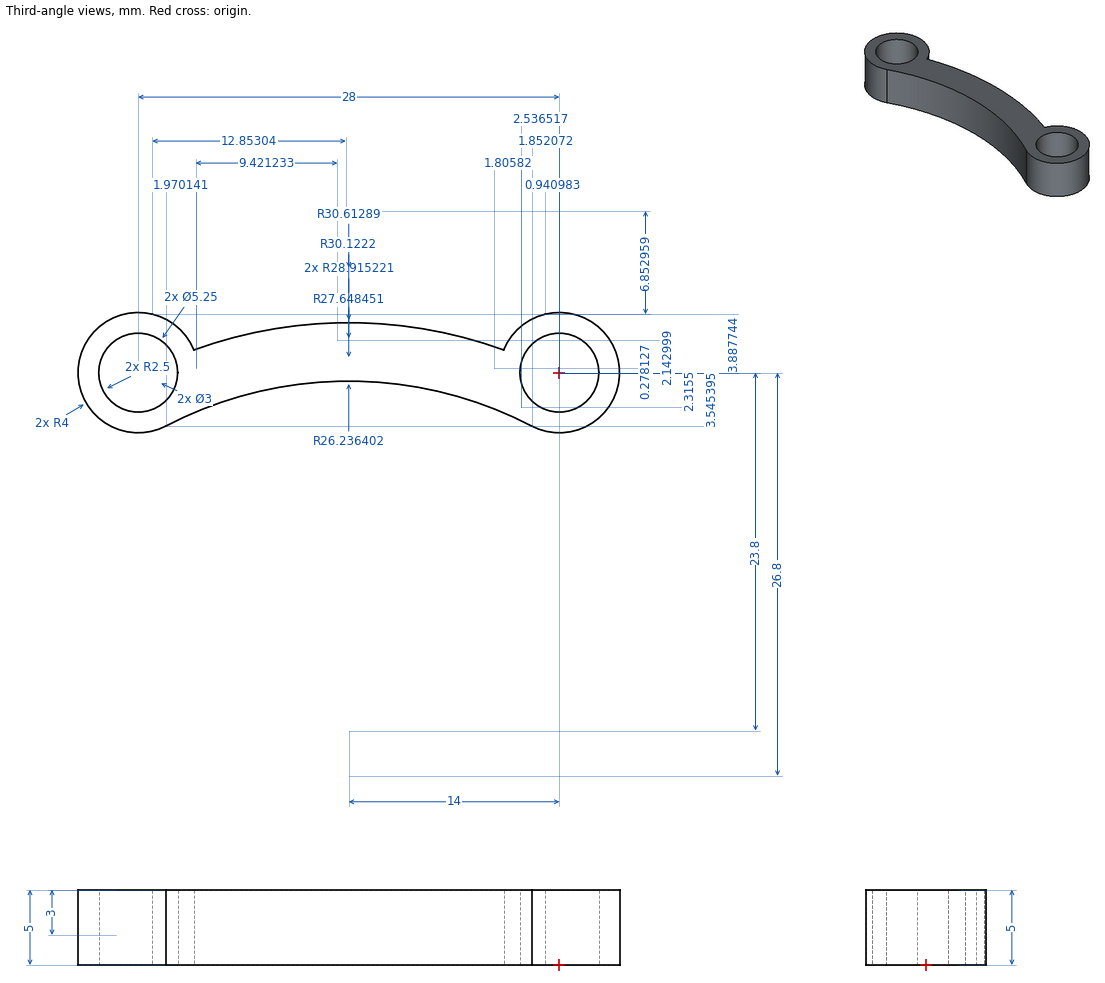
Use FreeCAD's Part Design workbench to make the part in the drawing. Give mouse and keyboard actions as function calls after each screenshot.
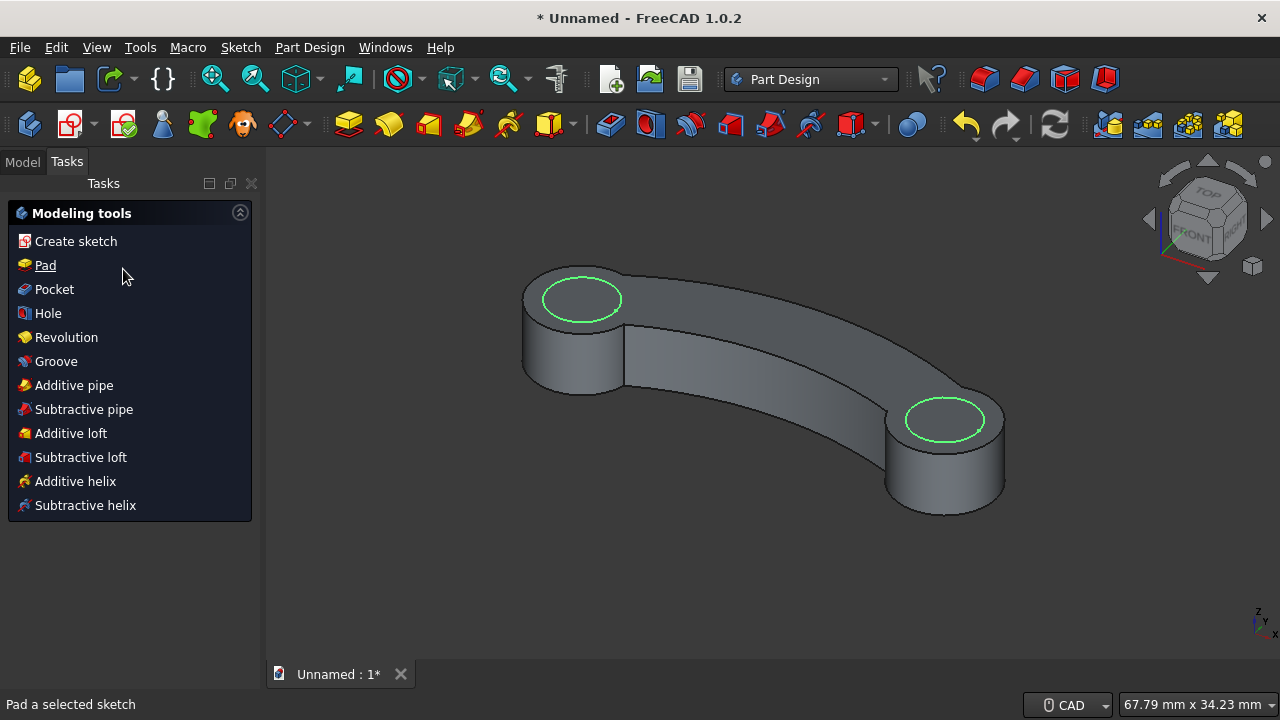
click(612, 124)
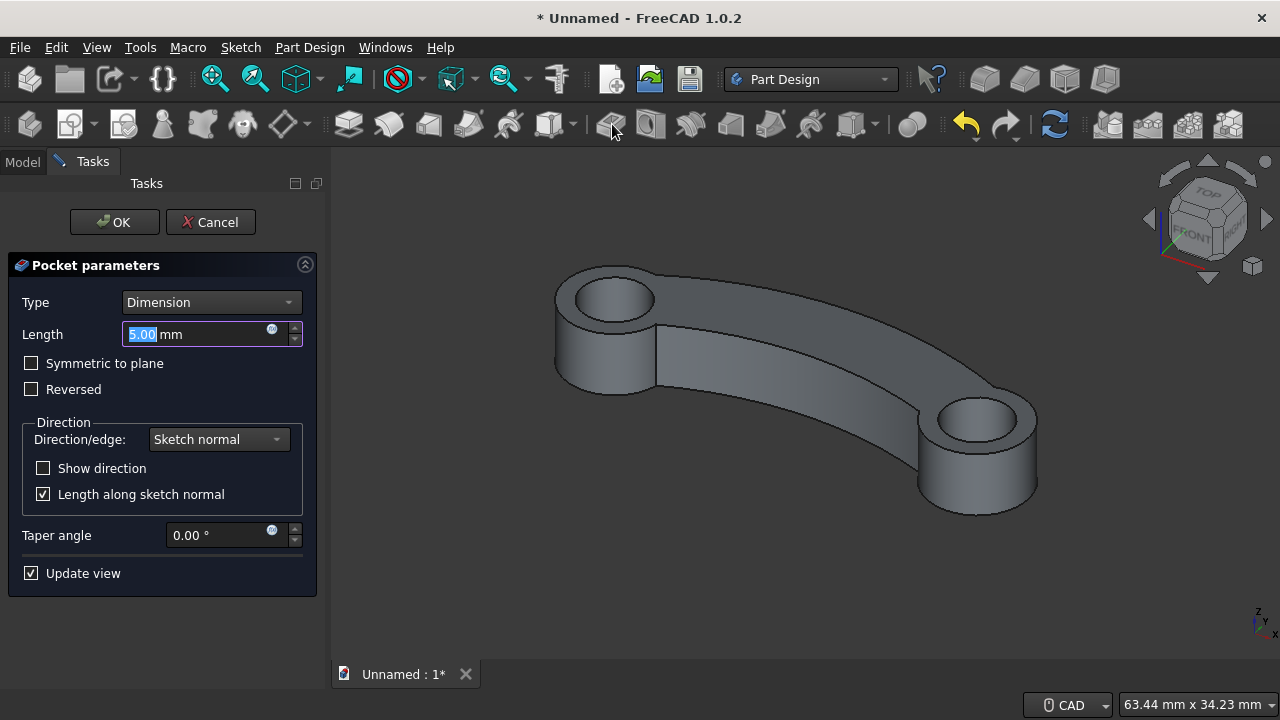
click(212, 302)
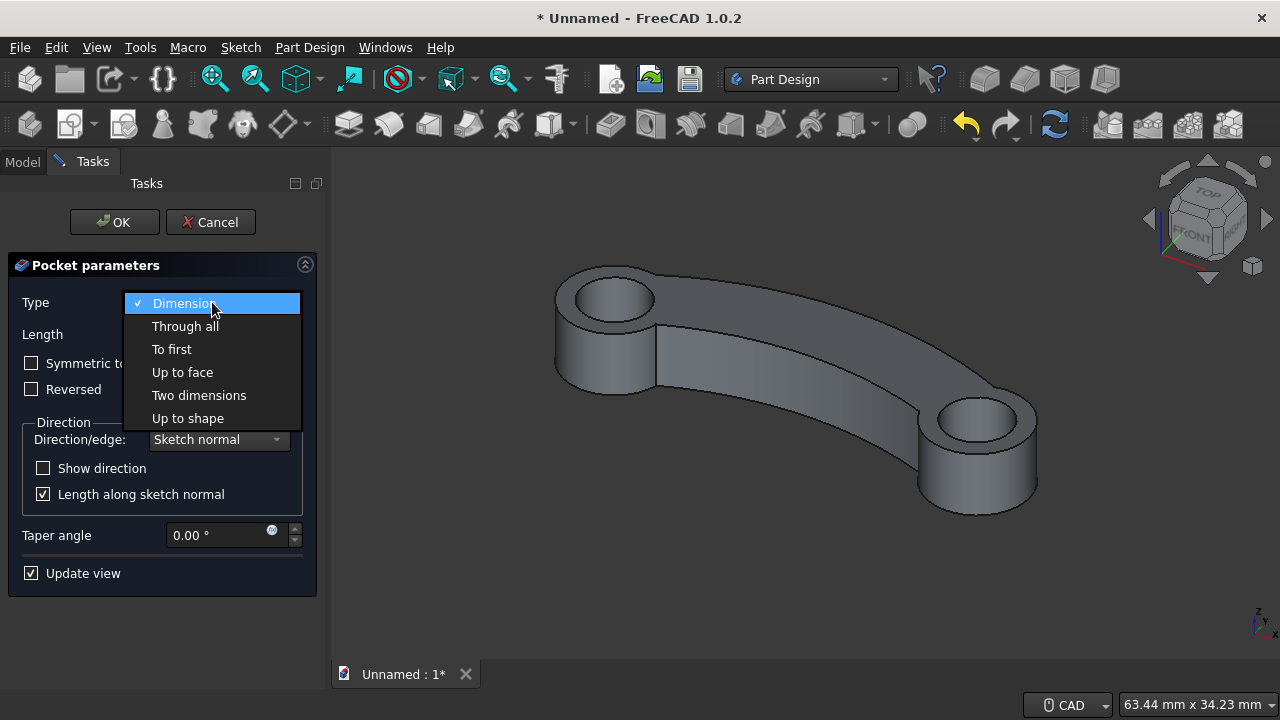
click(212, 326)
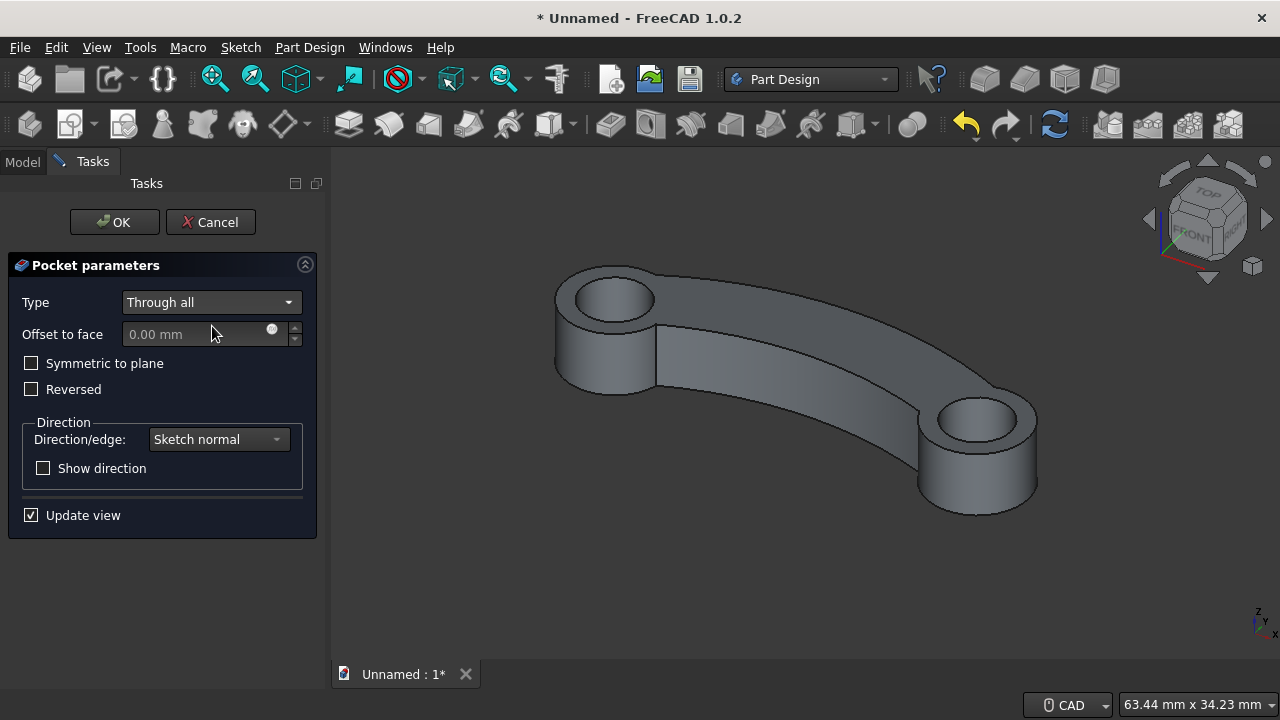
click(115, 222)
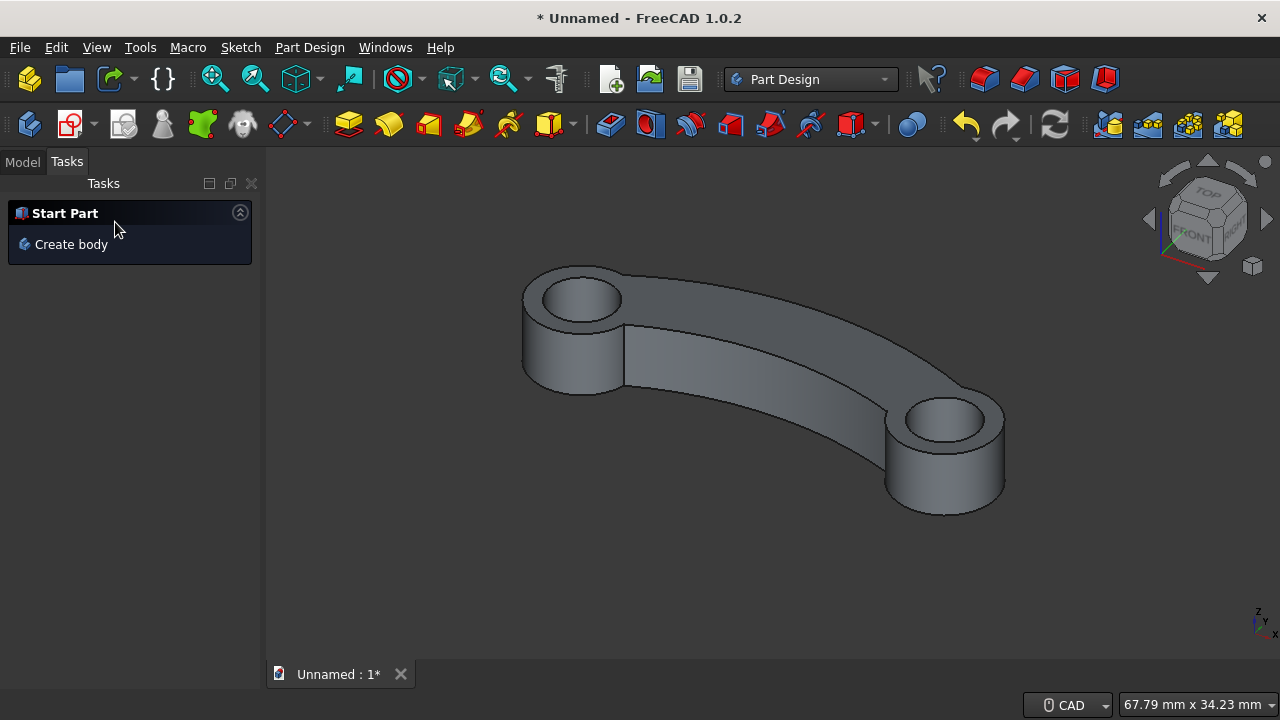
click(852, 359)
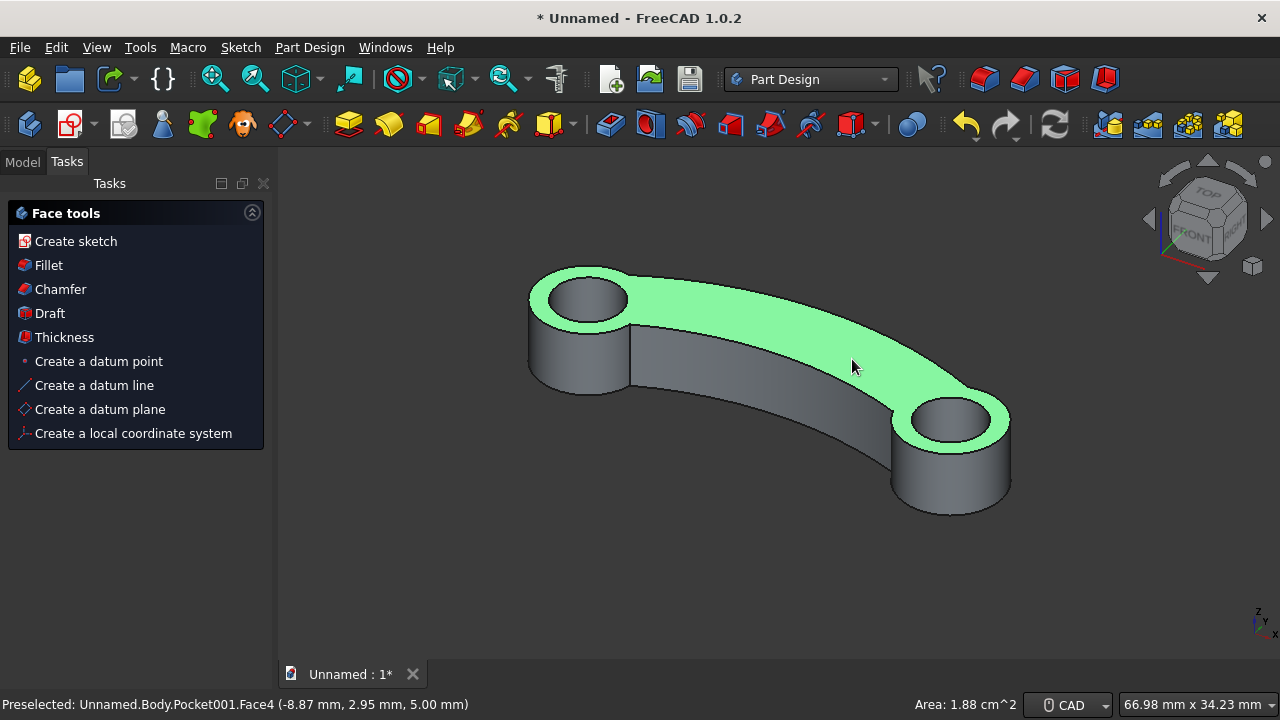
click(70, 124)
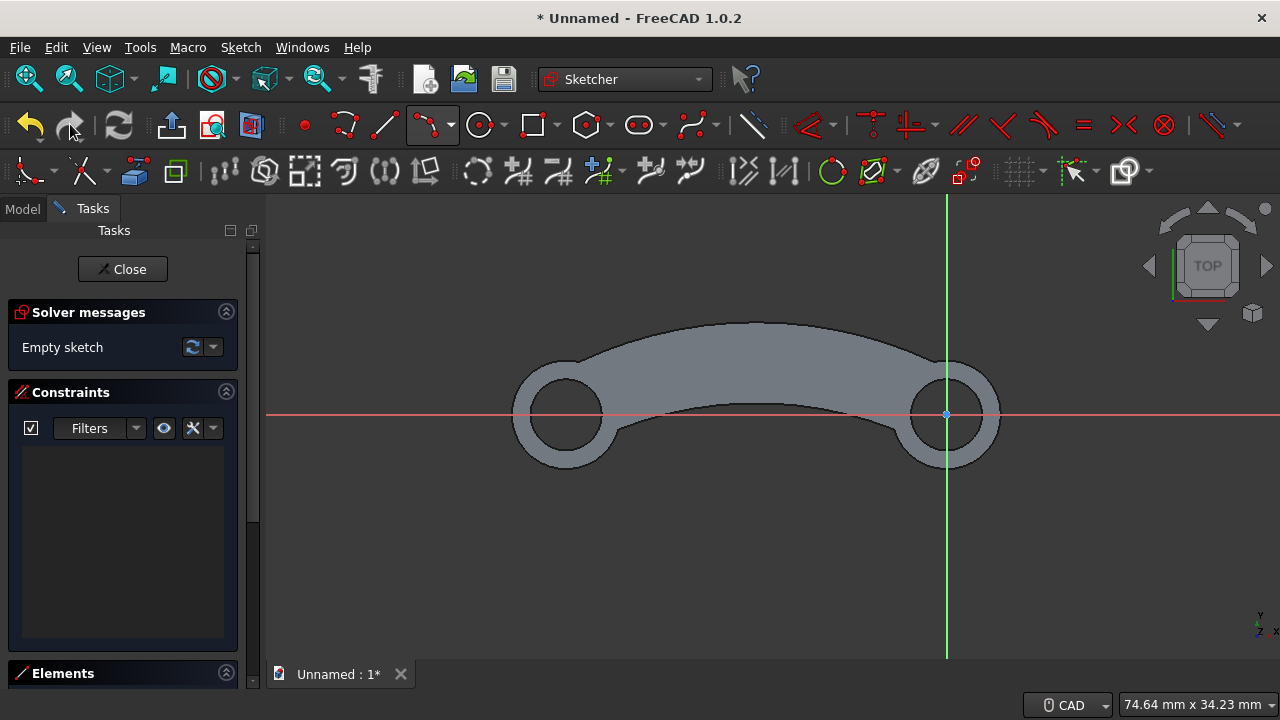
scroll(881, 222, up, 2)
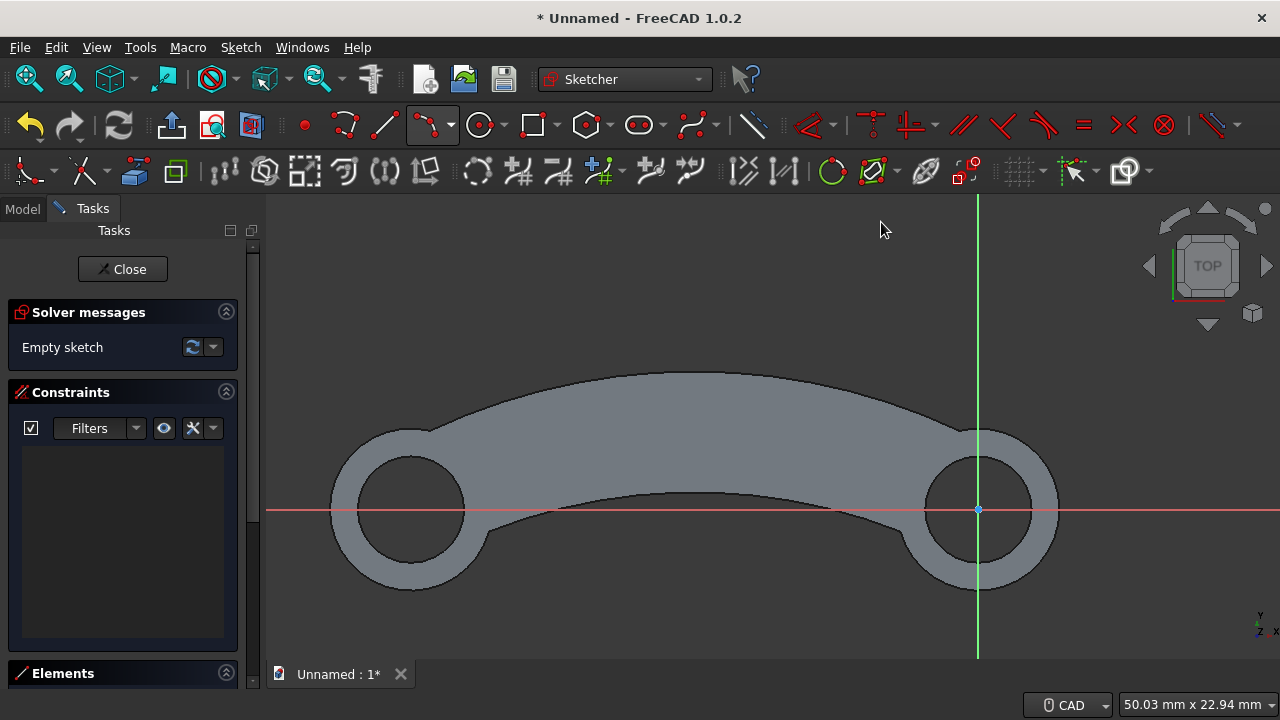
click(346, 126)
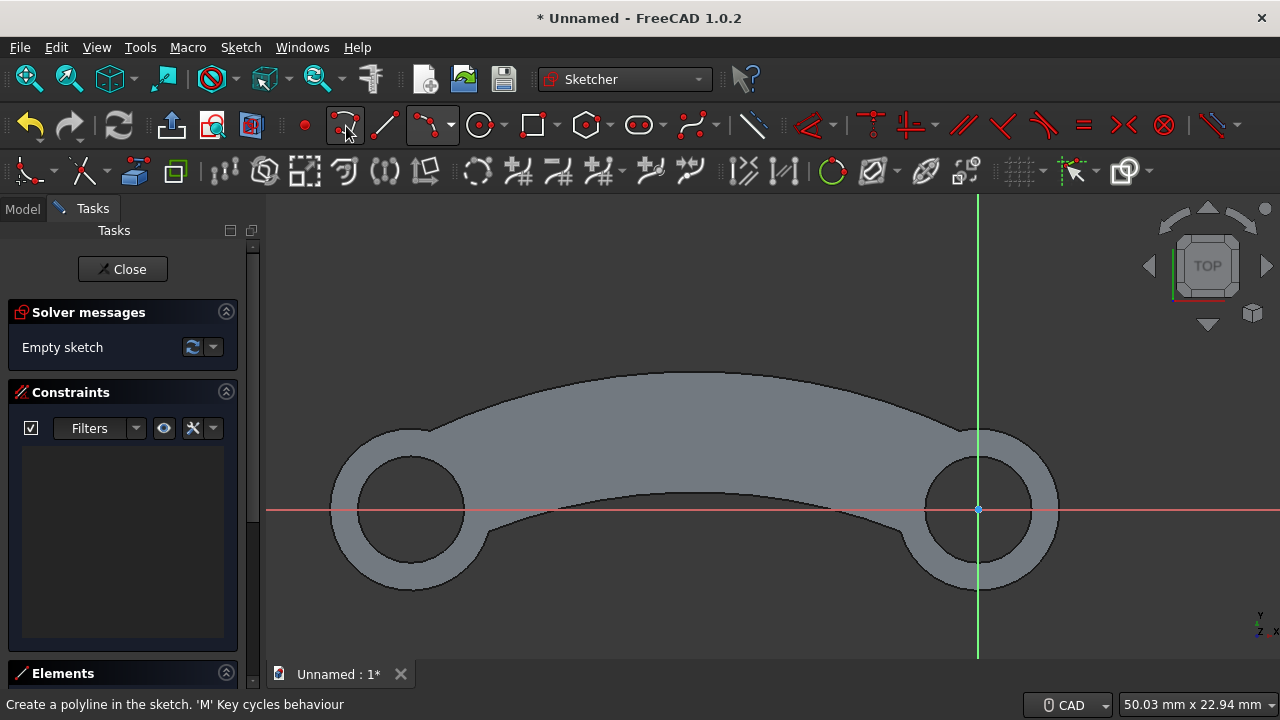
click(959, 431)
click(691, 292)
click(430, 431)
right_click(430, 431)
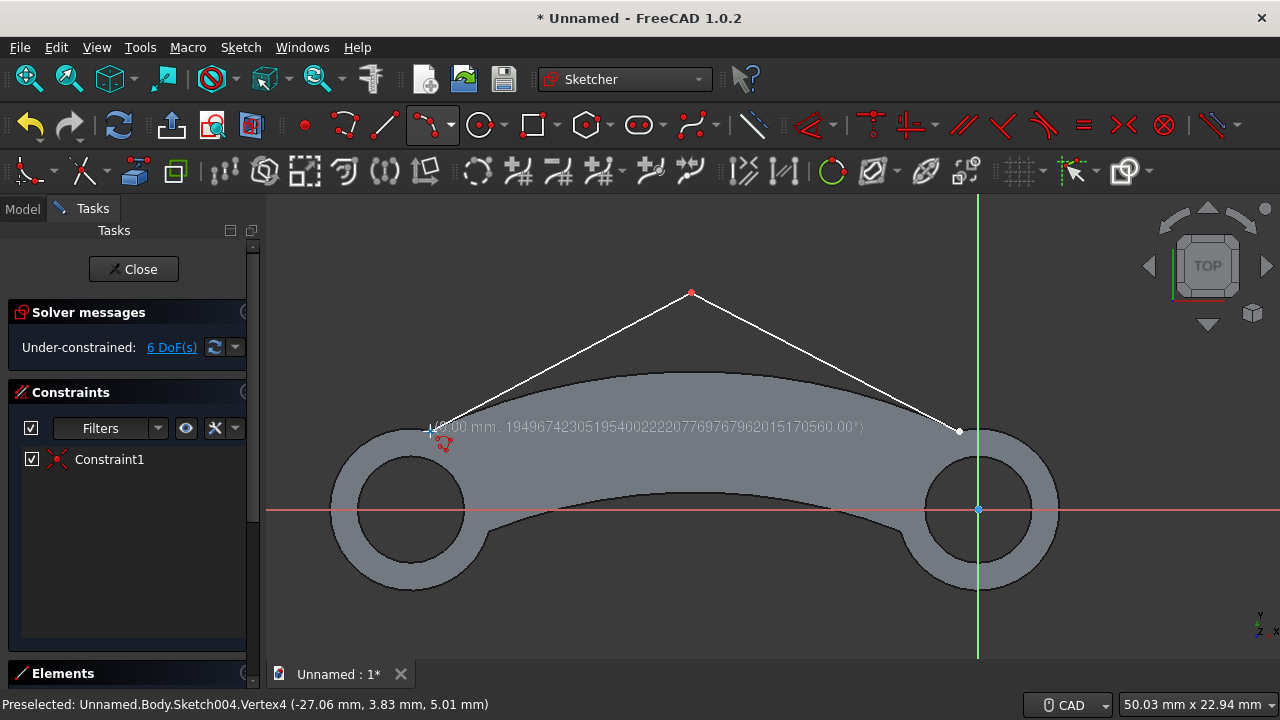
click(426, 126)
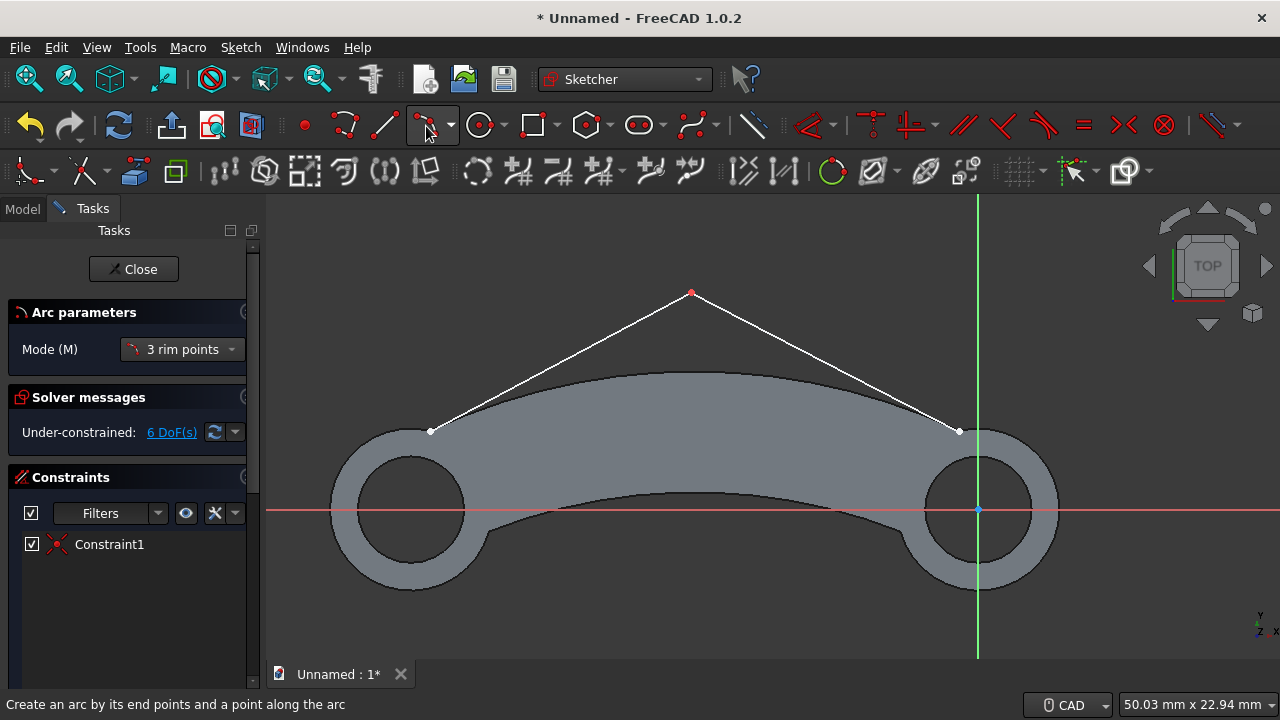
click(430, 432)
click(486, 479)